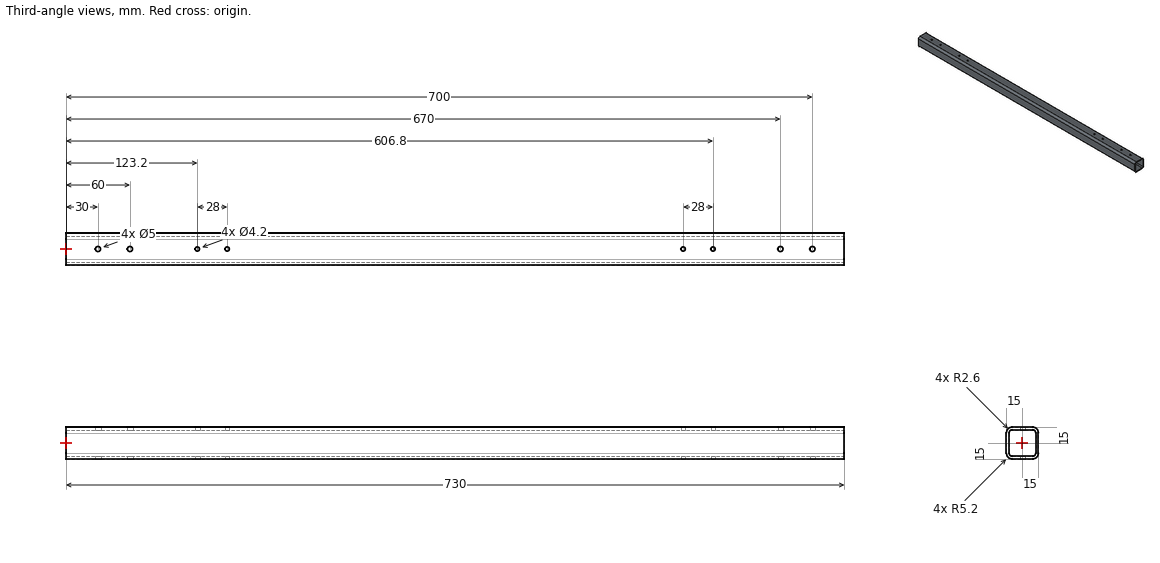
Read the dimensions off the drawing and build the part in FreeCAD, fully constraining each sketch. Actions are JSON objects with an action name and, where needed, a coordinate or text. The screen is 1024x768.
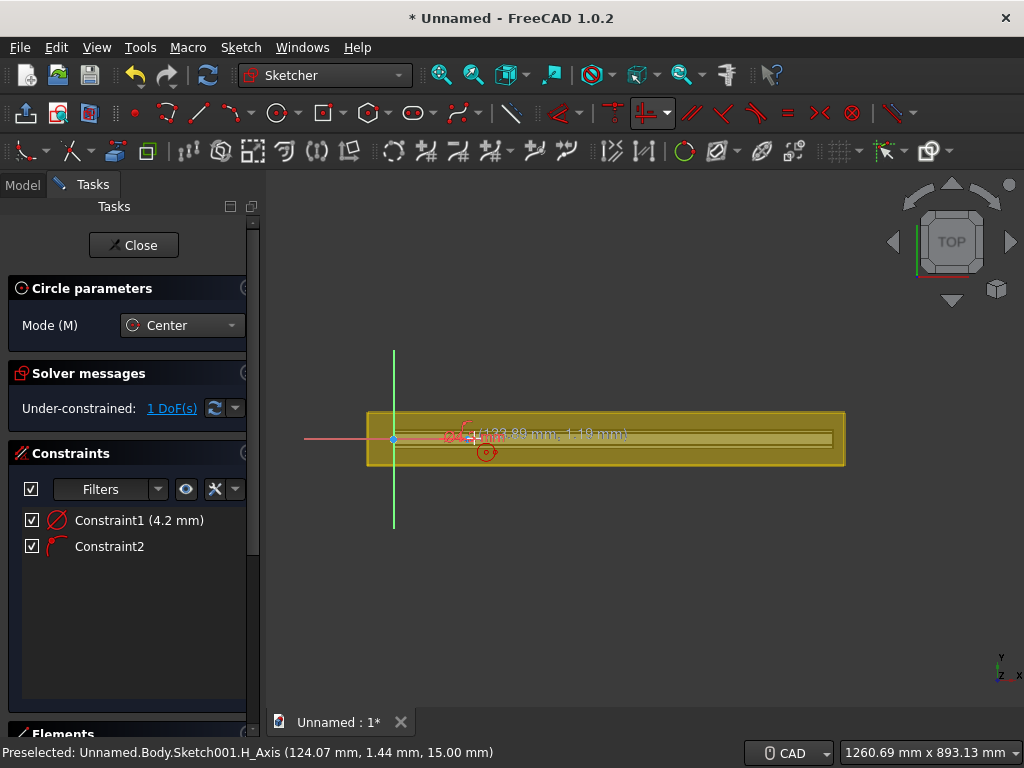
{"action": "left_click", "coordinate": [485, 439]}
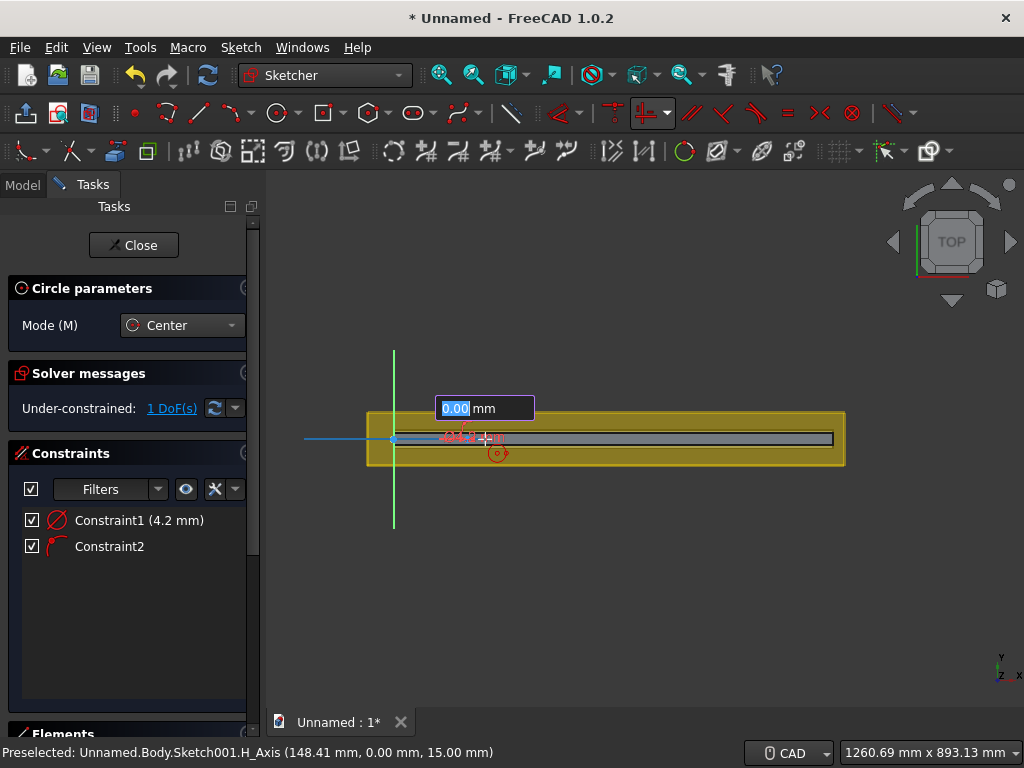
{"action": "scroll", "coordinate": [484, 440], "scroll_direction": "up", "scroll_amount": 13}
{"action": "mouse_move", "coordinate": [484, 439]}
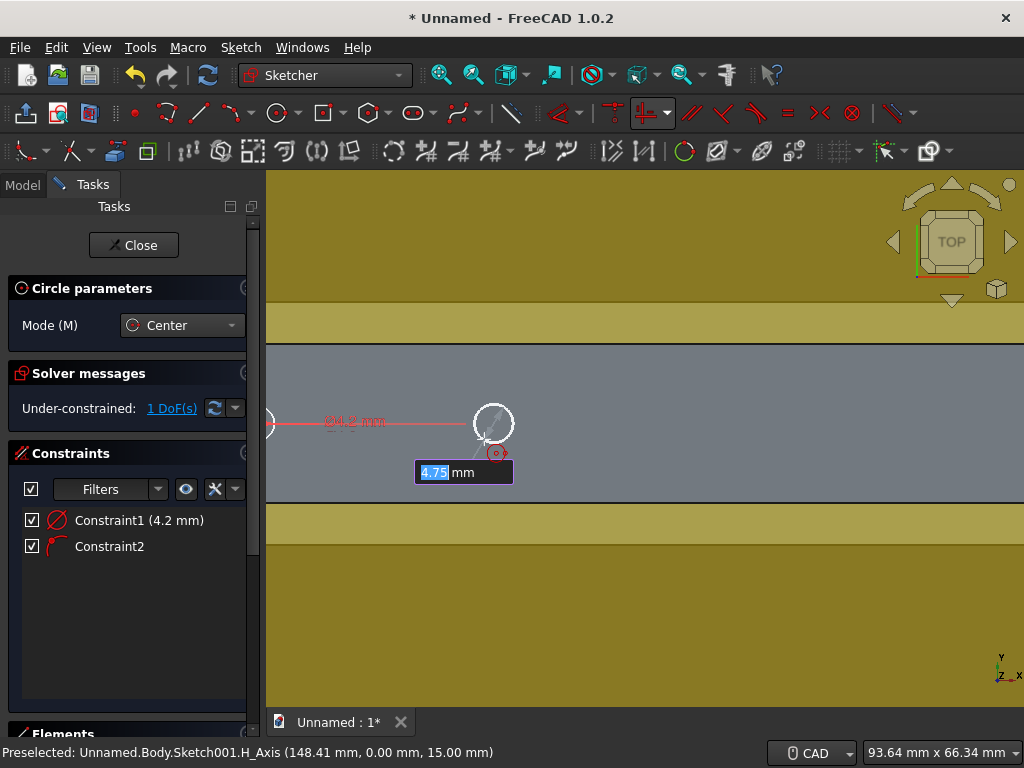
{"action": "type", "text": "4.2"}
{"action": "key", "text": "Return"}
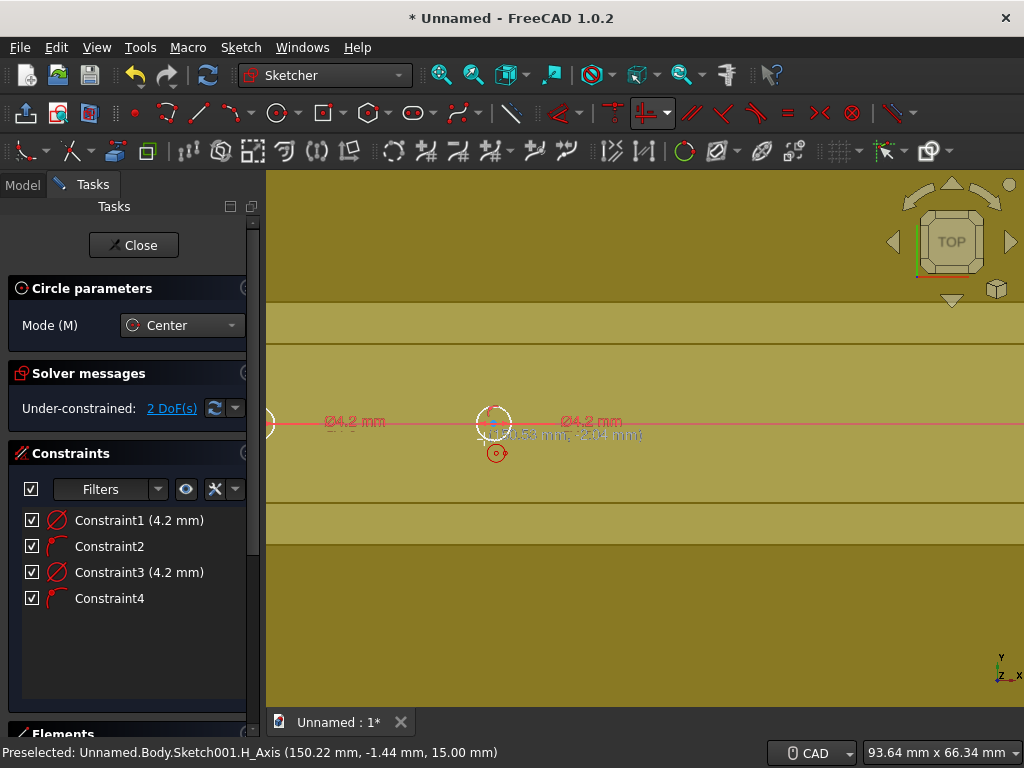
{"action": "scroll", "coordinate": [484, 440], "scroll_direction": "down", "scroll_amount": 13}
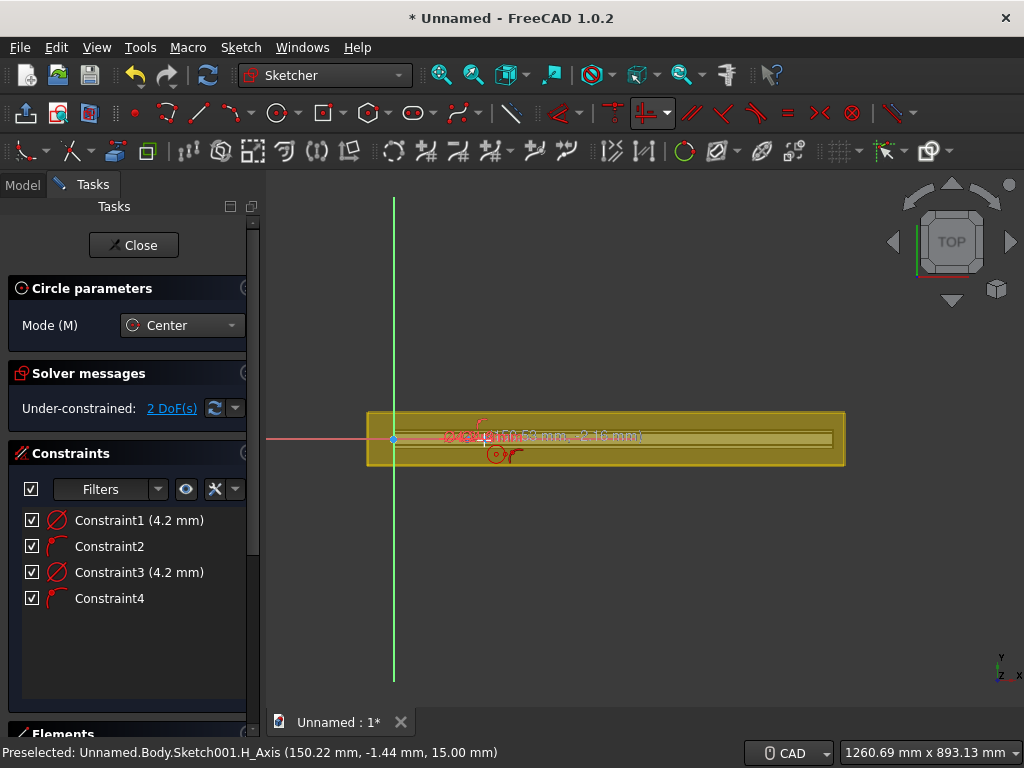
{"action": "scroll", "coordinate": [759, 439], "scroll_direction": "up", "scroll_amount": 15}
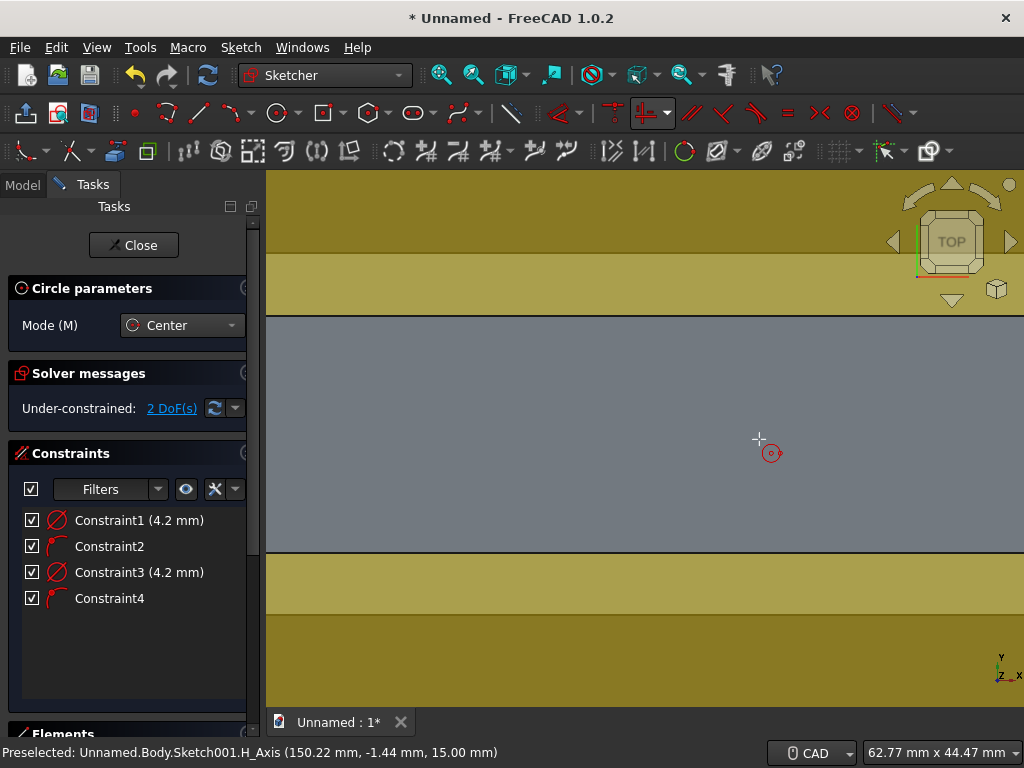
{"action": "scroll", "coordinate": [759, 439], "scroll_direction": "down", "scroll_amount": 15}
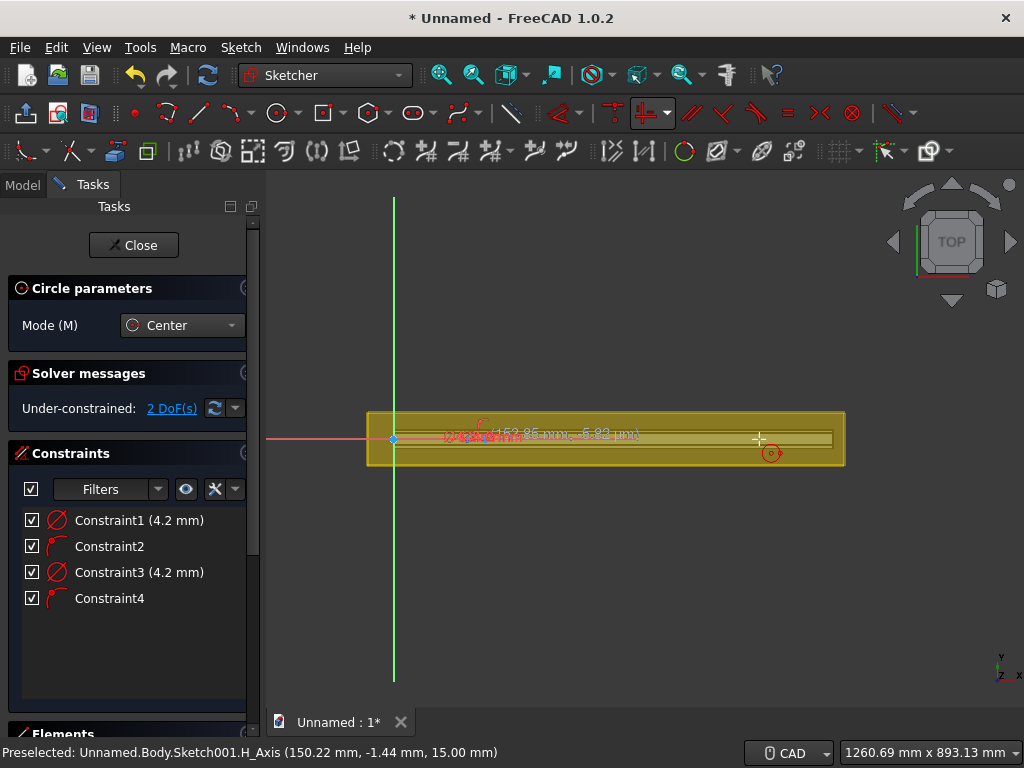
{"action": "left_click", "coordinate": [759, 439]}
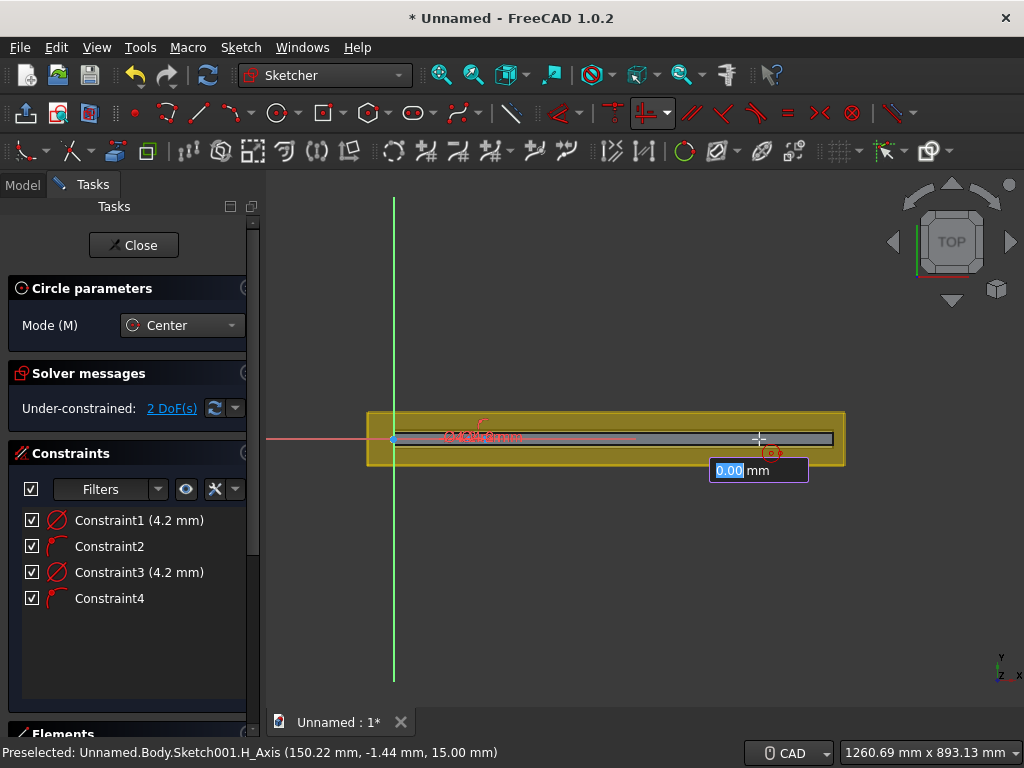
{"action": "scroll", "coordinate": [759, 438], "scroll_direction": "up", "scroll_amount": 13}
{"action": "mouse_move", "coordinate": [751, 433]}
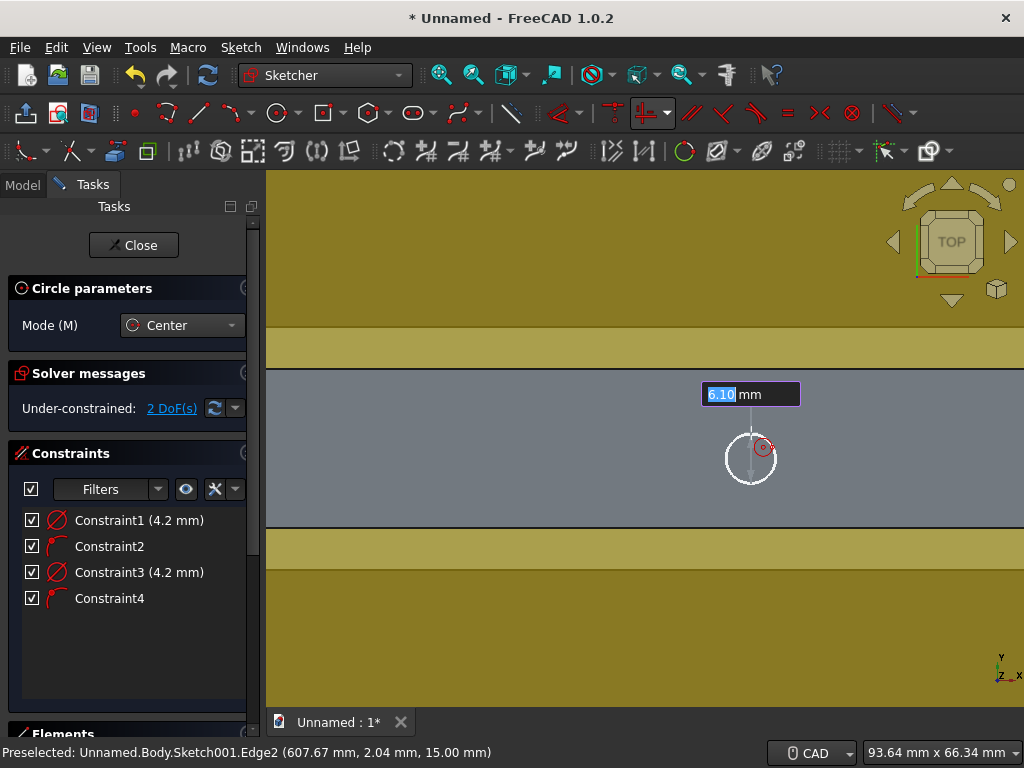
{"action": "type", "text": "4.2"}
{"action": "key", "text": "Return"}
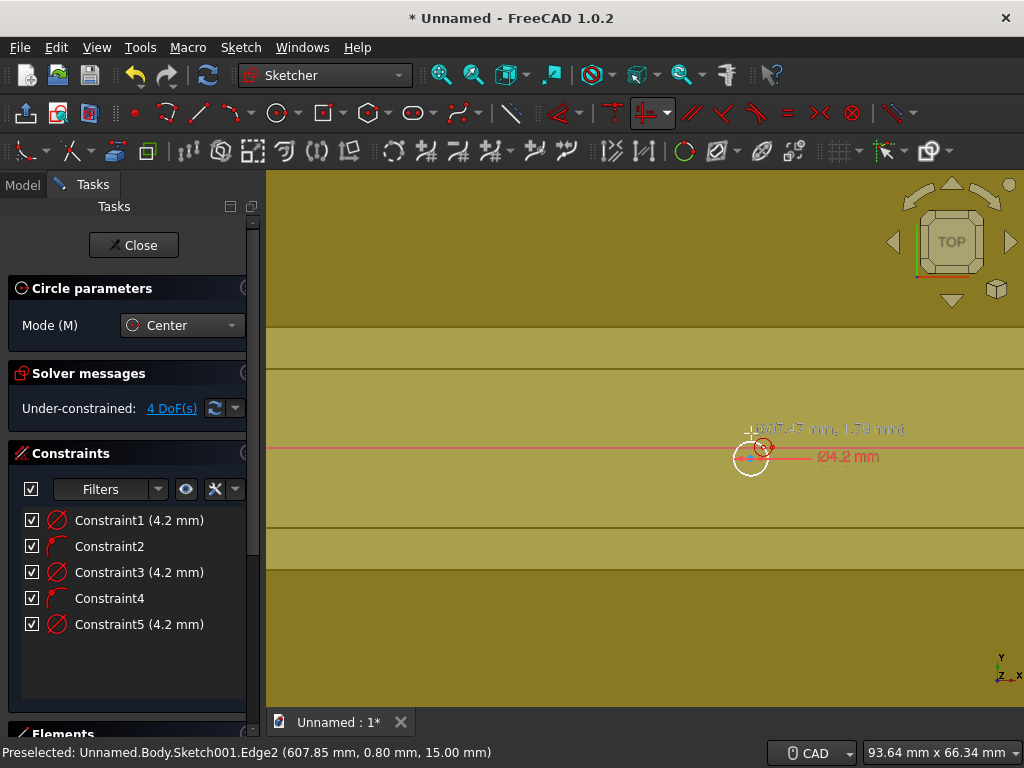
{"action": "scroll", "coordinate": [519, 448], "scroll_direction": "up", "scroll_amount": 2}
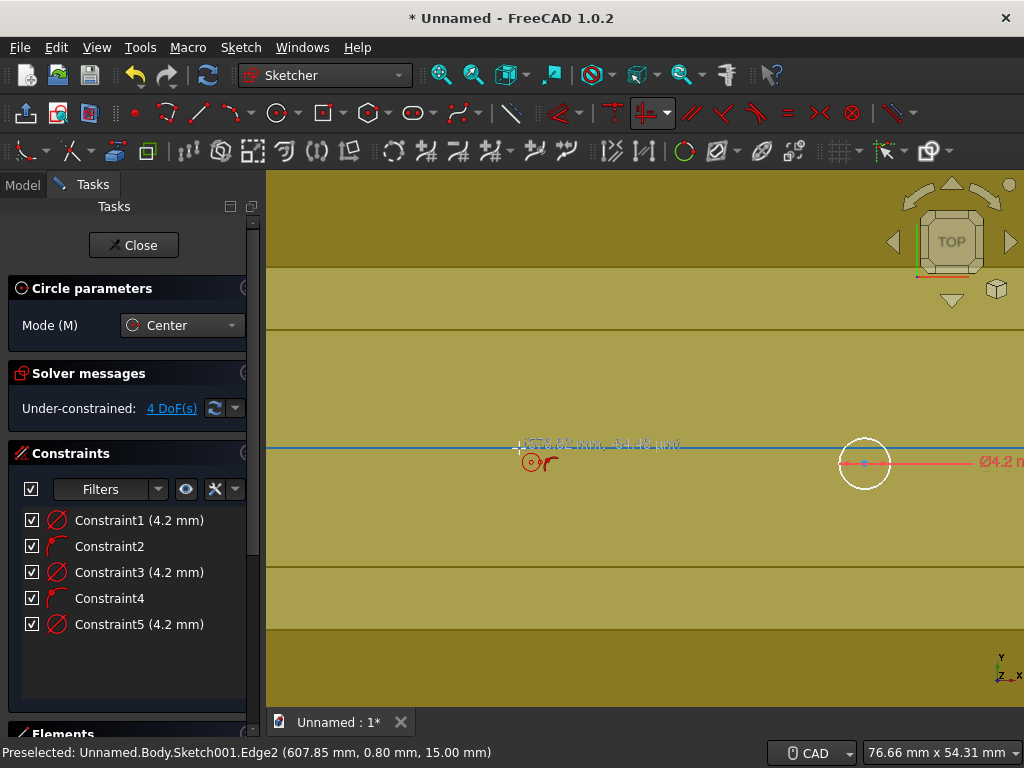
{"action": "scroll", "coordinate": [753, 438], "scroll_direction": "down", "scroll_amount": 15}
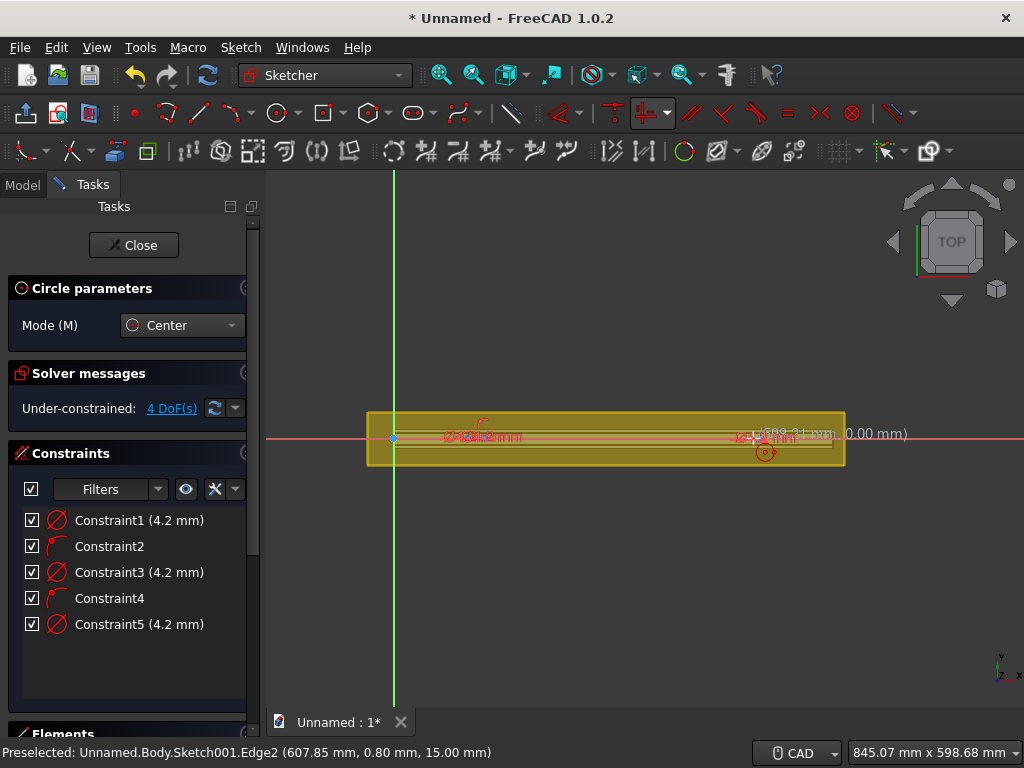
{"action": "left_click", "coordinate": [742, 439]}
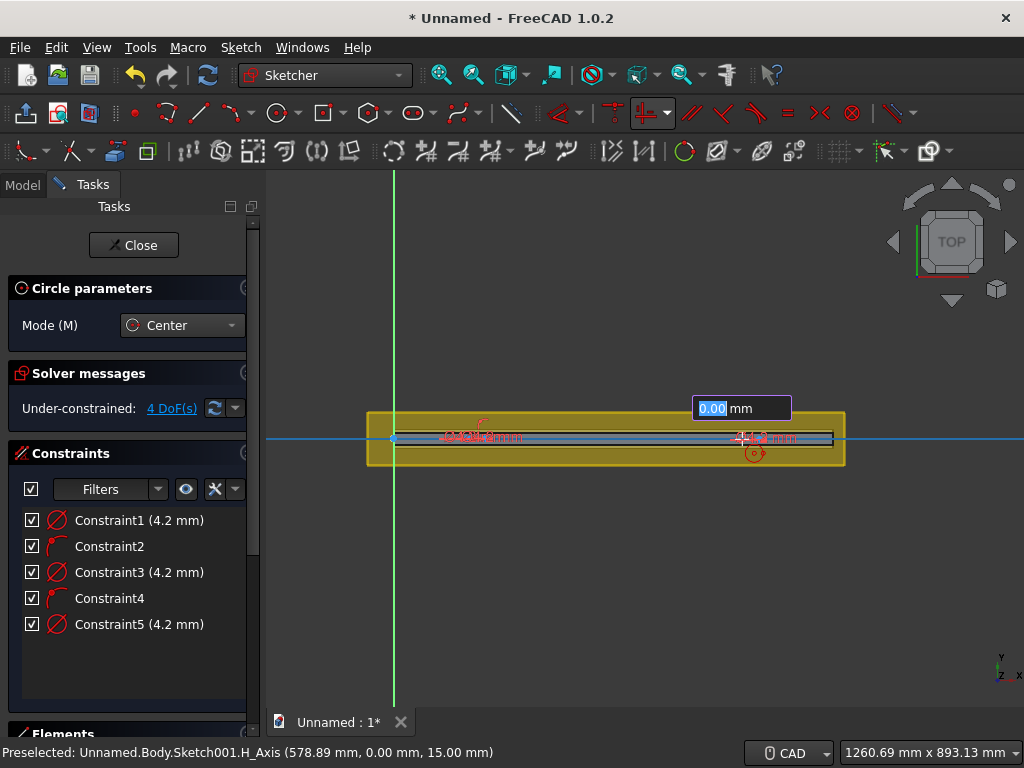
{"action": "scroll", "coordinate": [742, 438], "scroll_direction": "up", "scroll_amount": 13}
{"action": "mouse_move", "coordinate": [739, 429]}